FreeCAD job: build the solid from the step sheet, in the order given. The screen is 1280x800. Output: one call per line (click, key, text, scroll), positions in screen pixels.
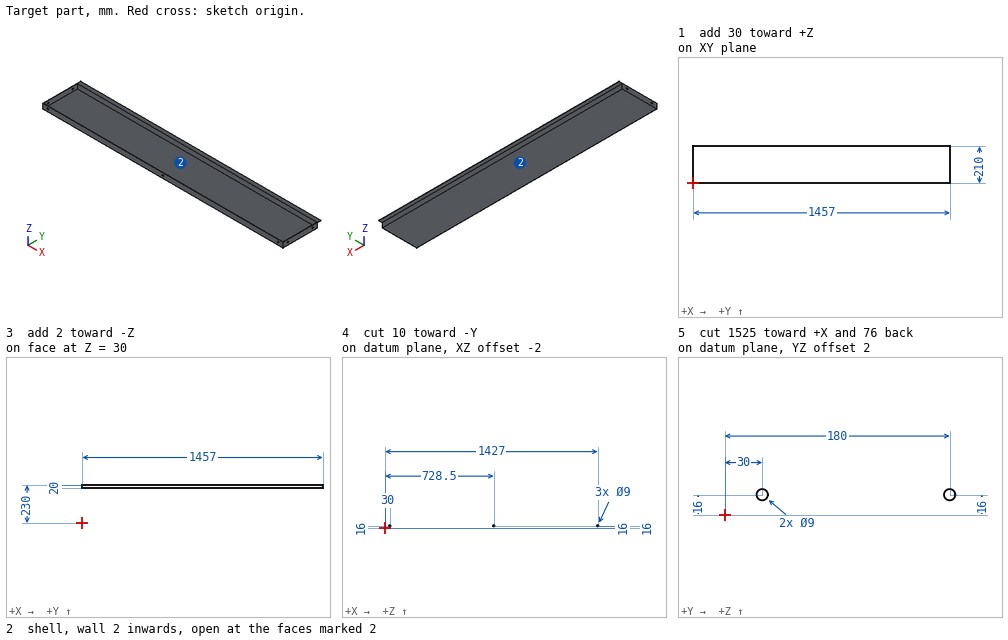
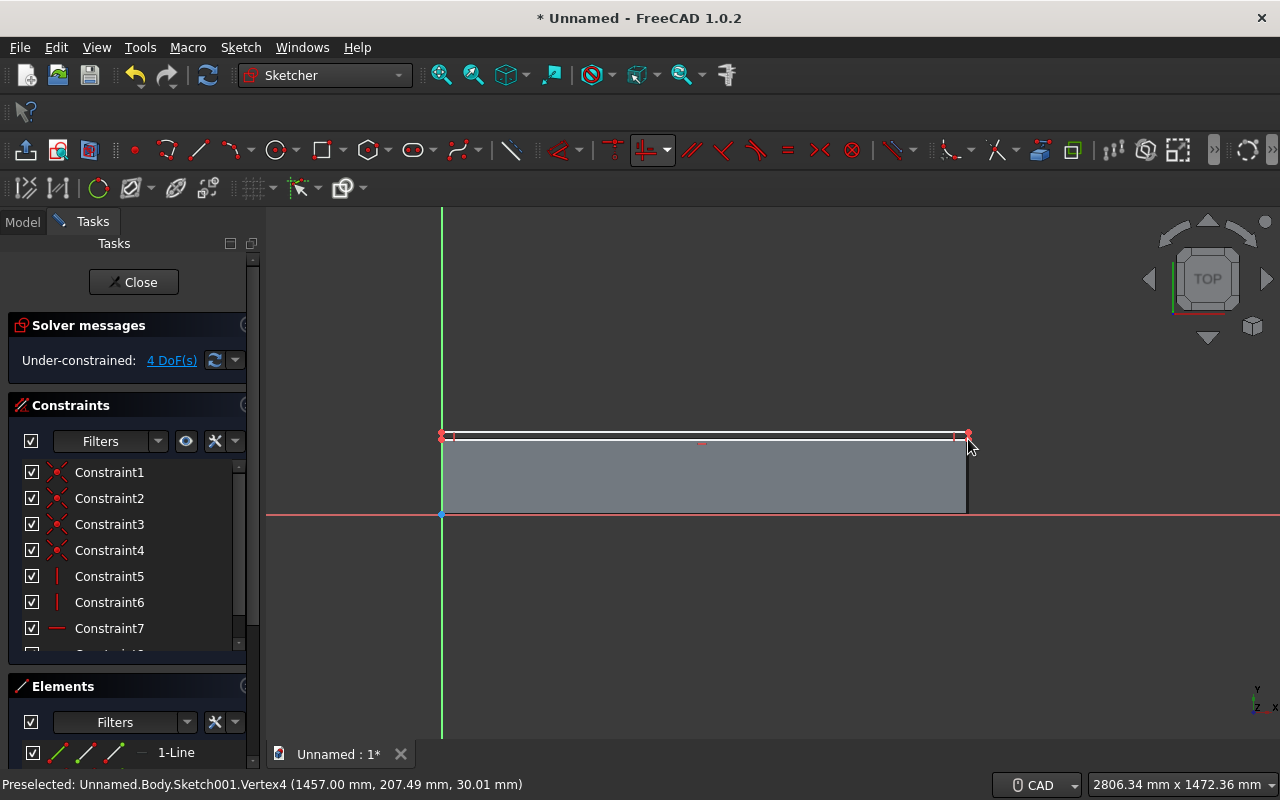
scroll(442, 432, up, 3)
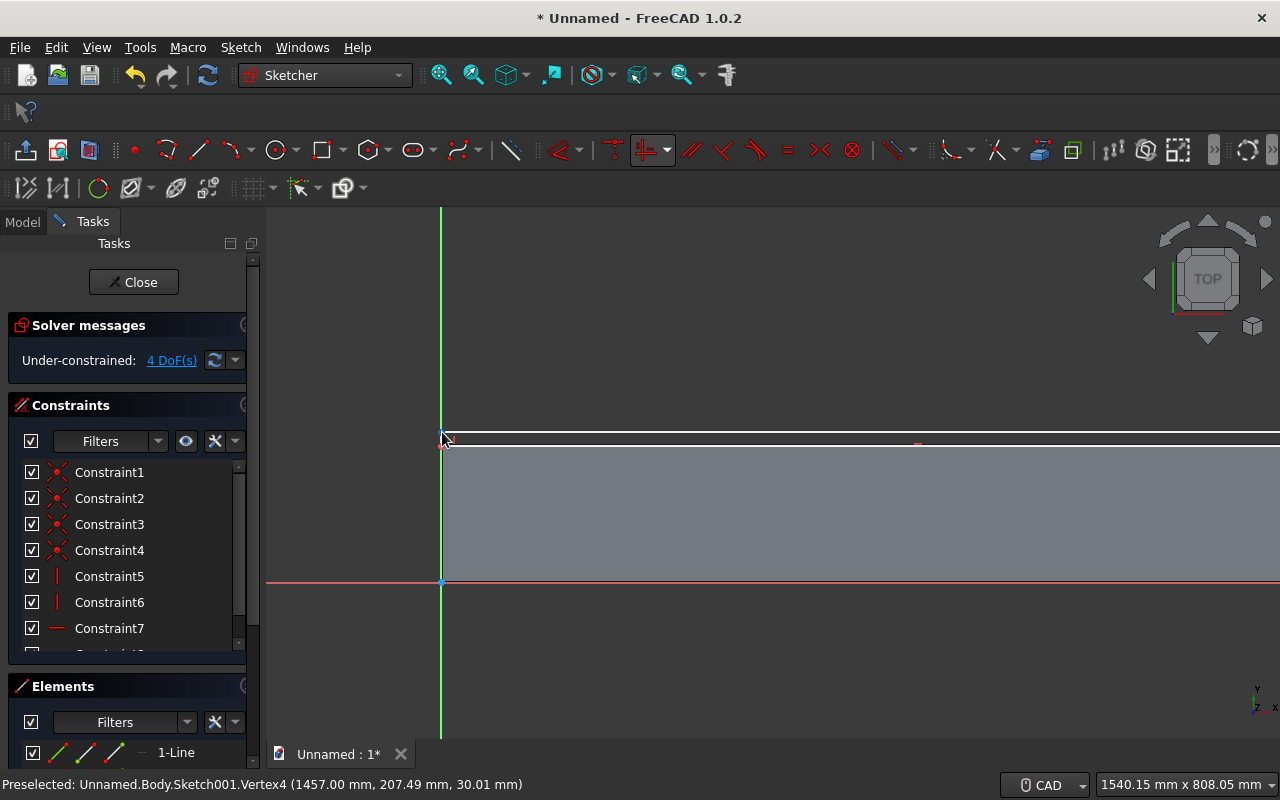
click(441, 432)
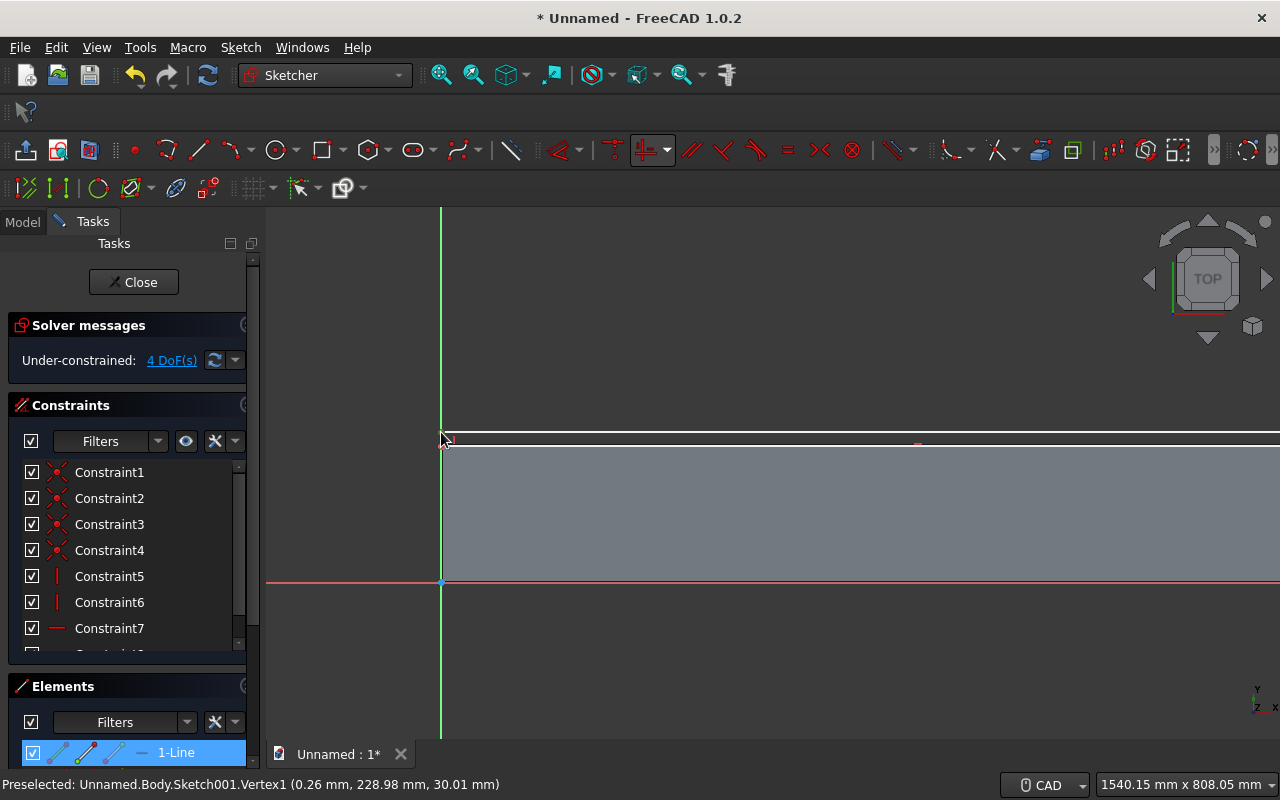
click(441, 677)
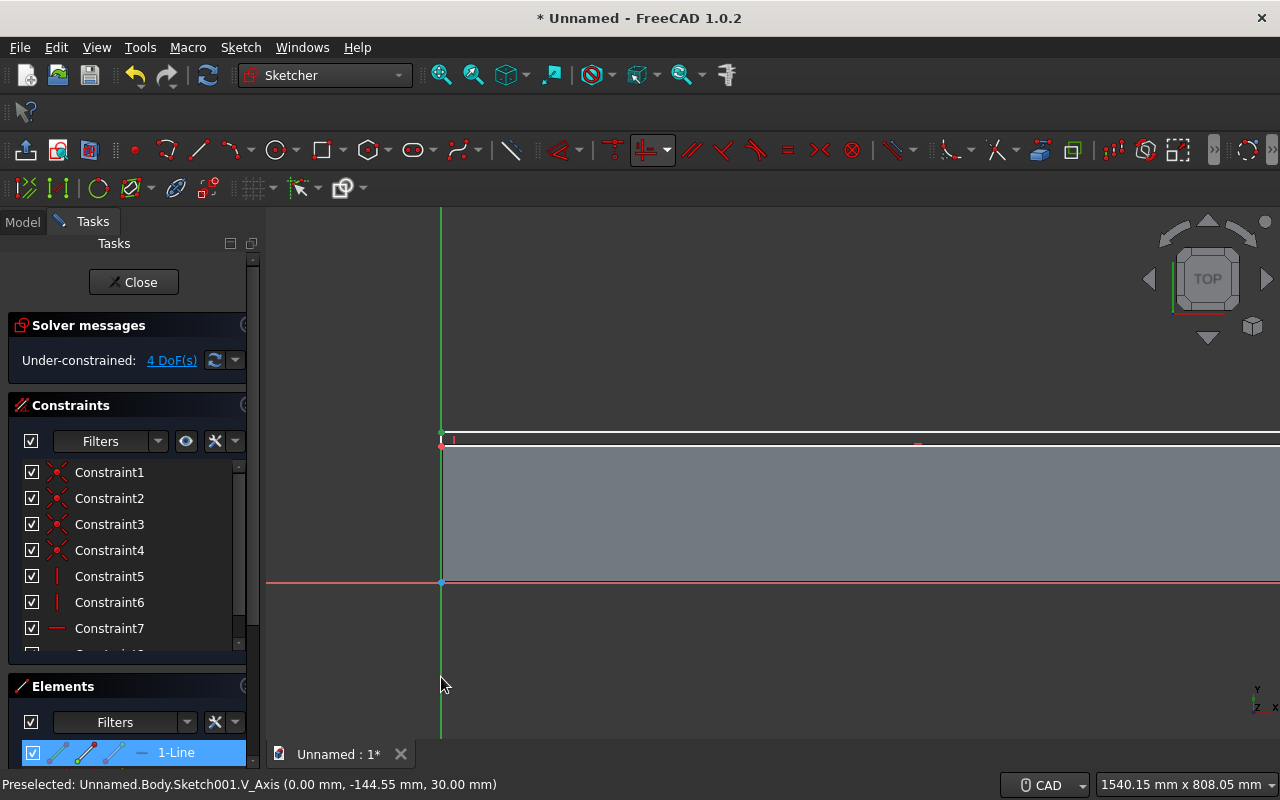
click(614, 150)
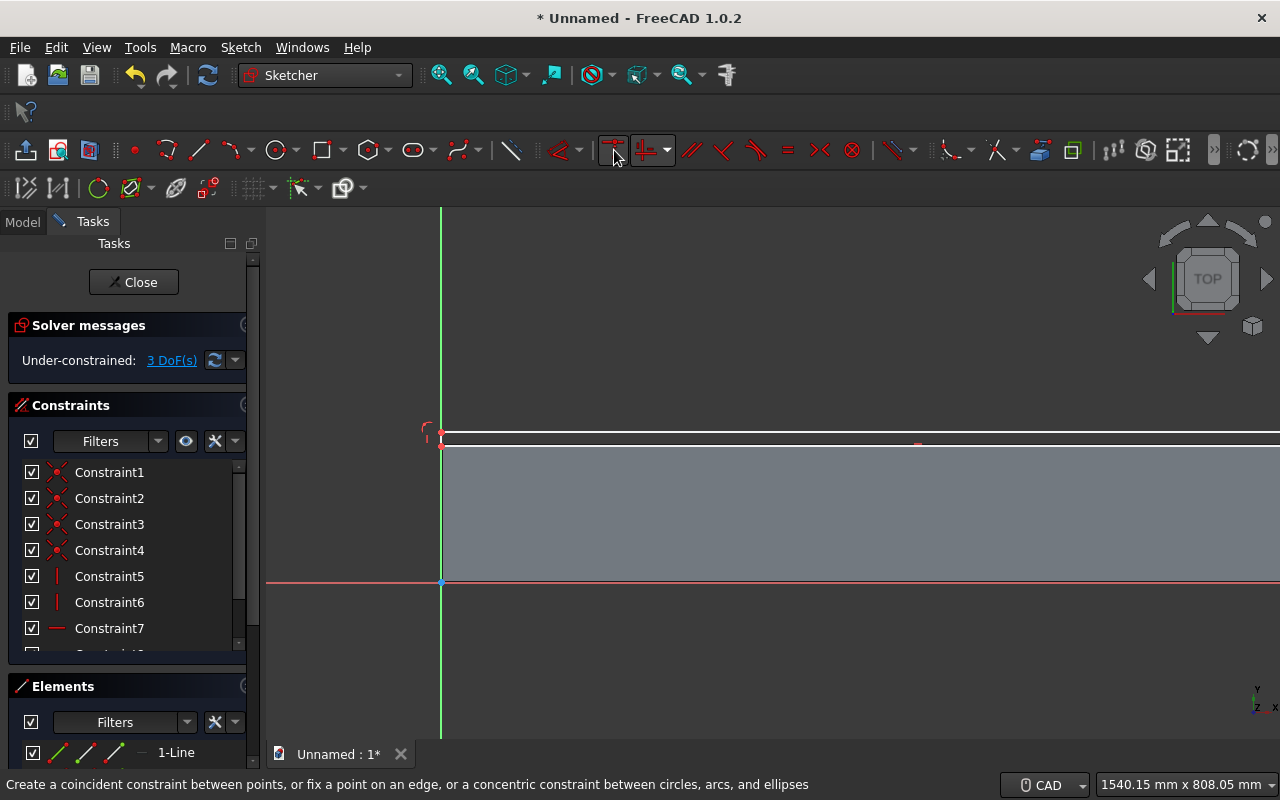
click(558, 150)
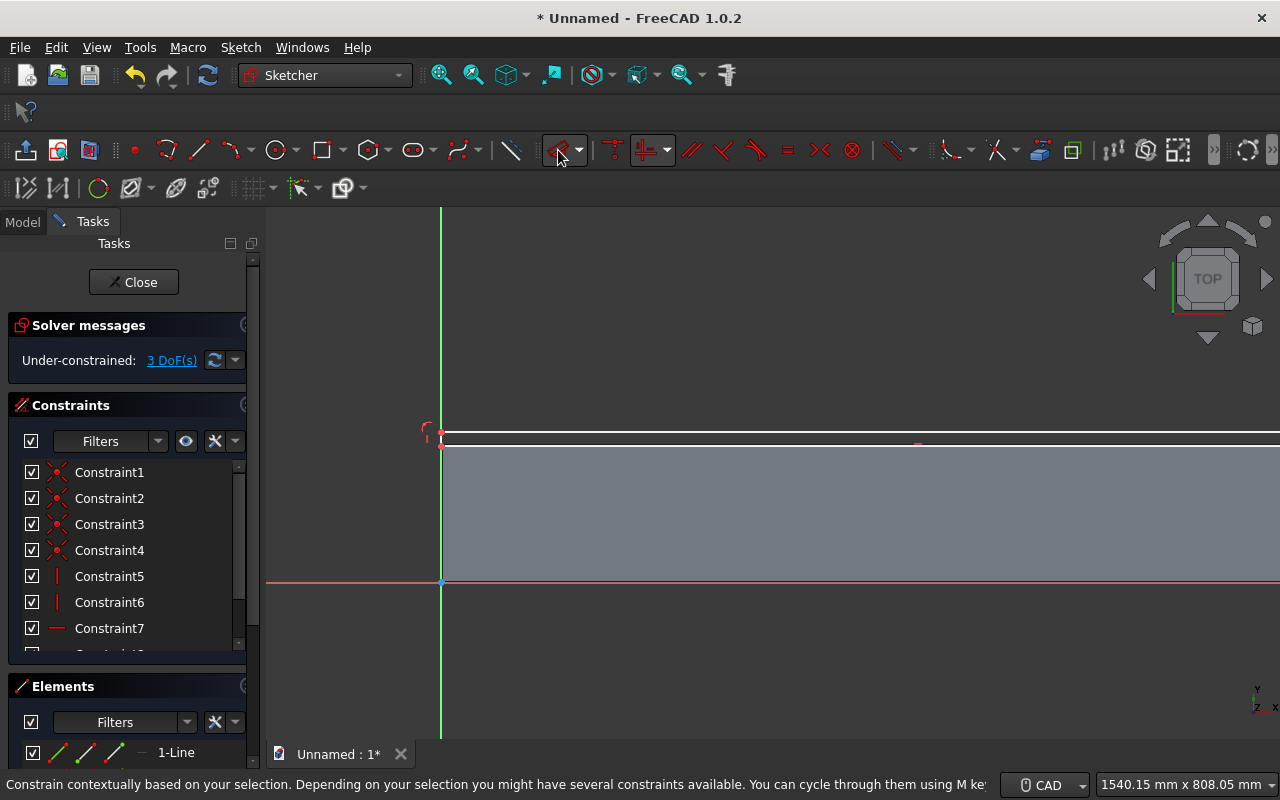
scroll(441, 439, up, 6)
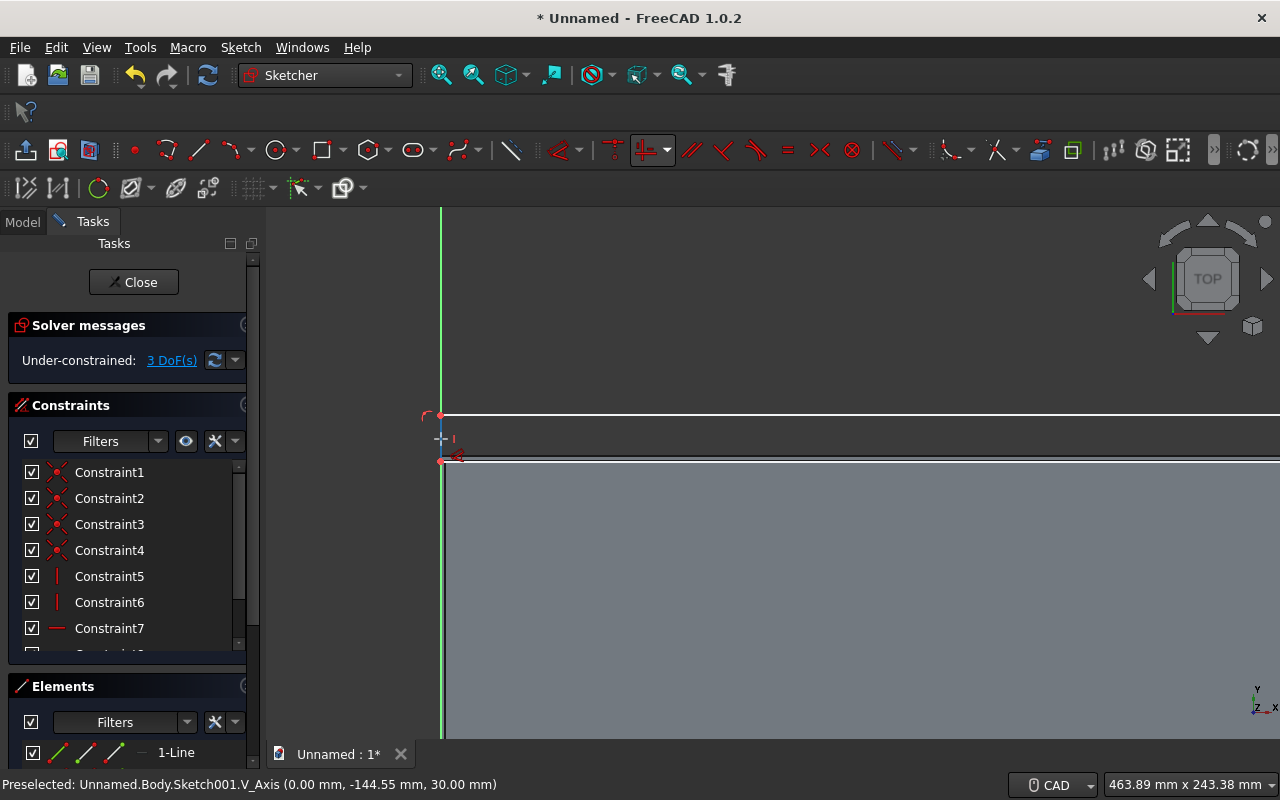
click(441, 438)
click(407, 438)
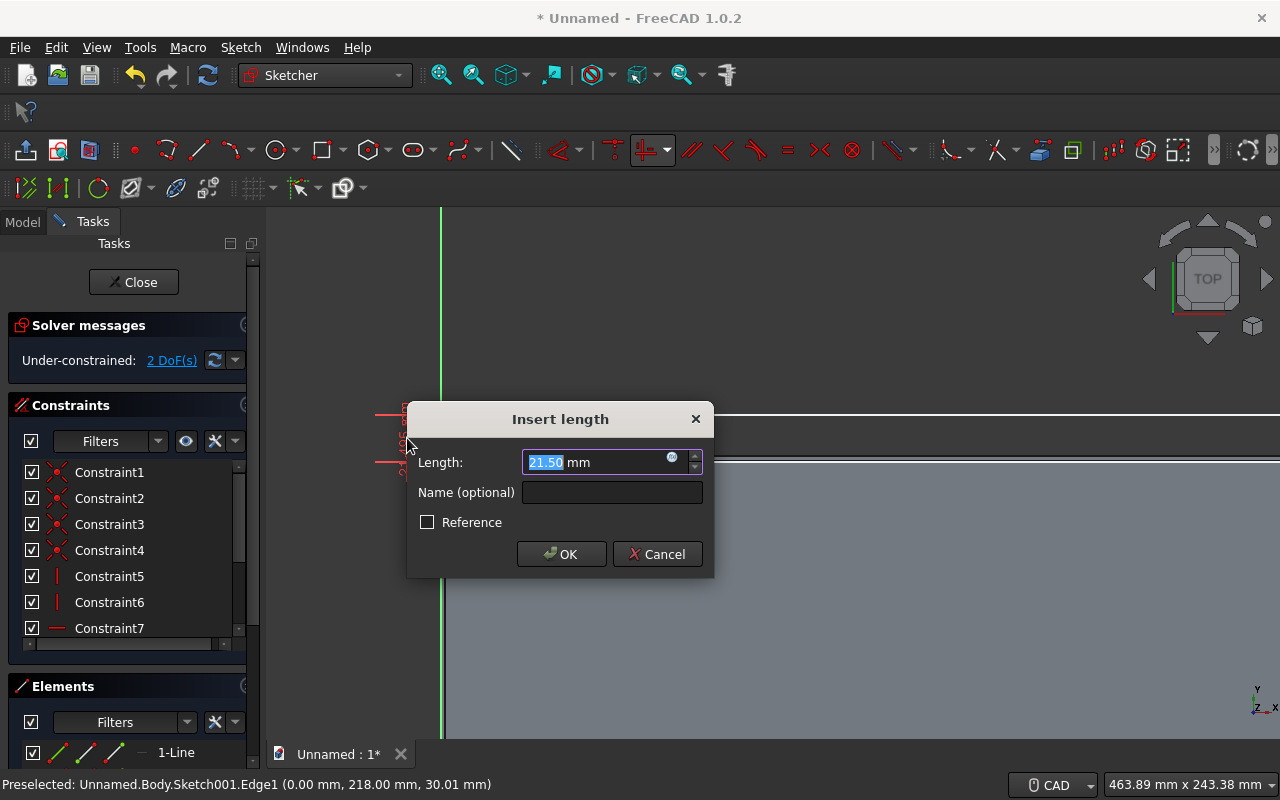
text(20)
key(Return)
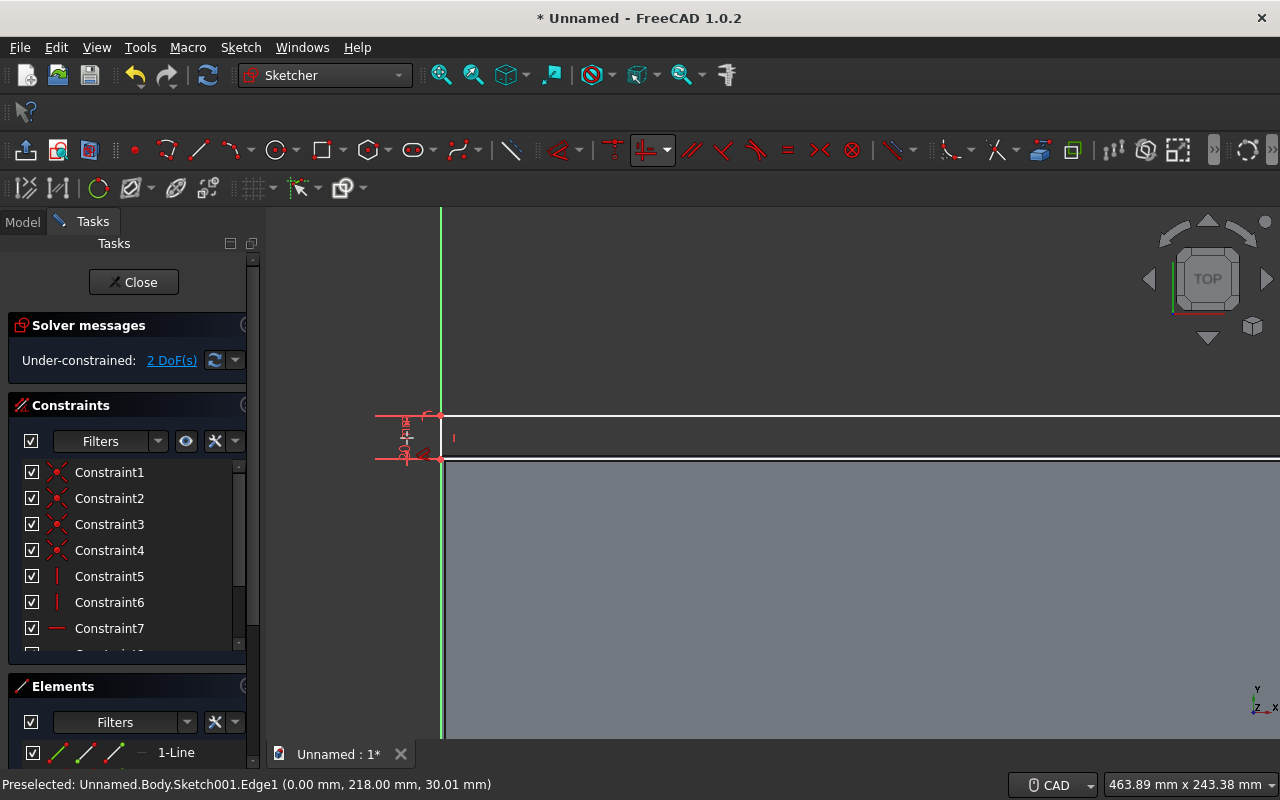
scroll(441, 435, down, 9)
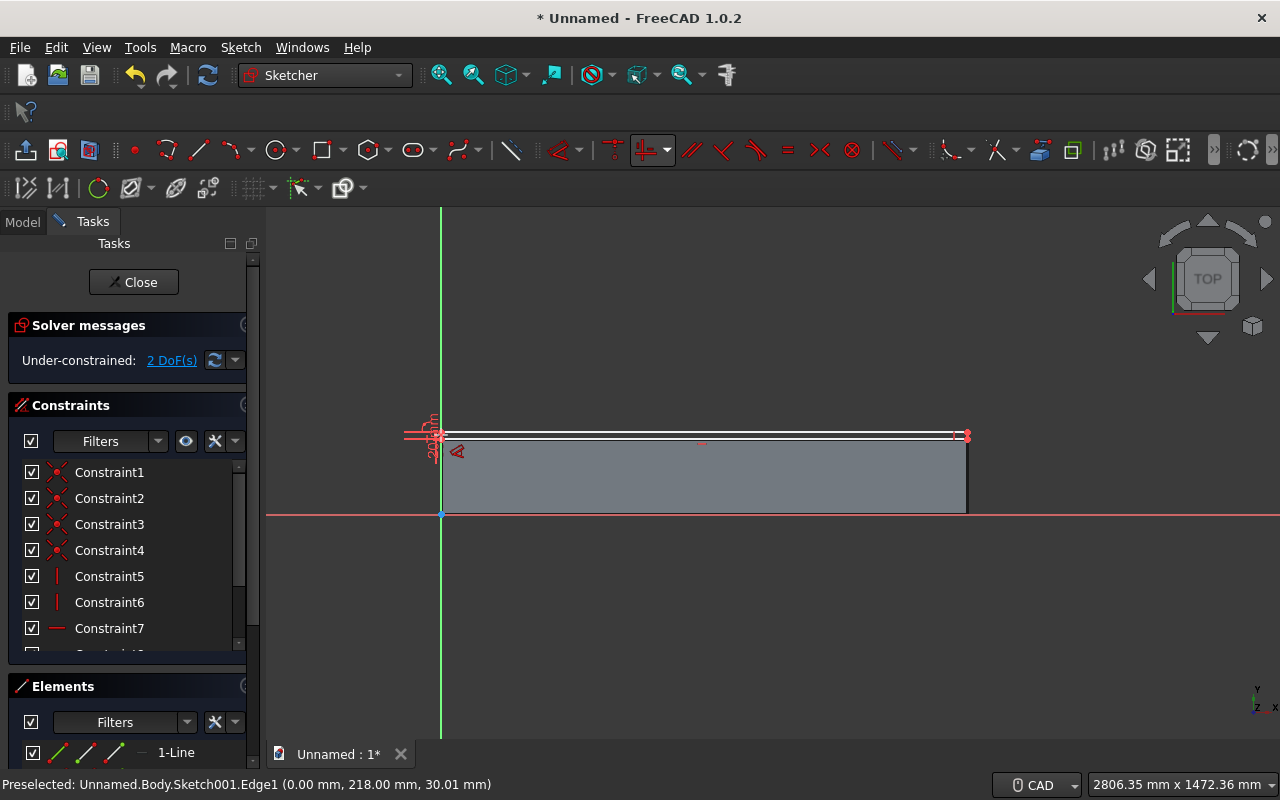
scroll(546, 439, up, 4)